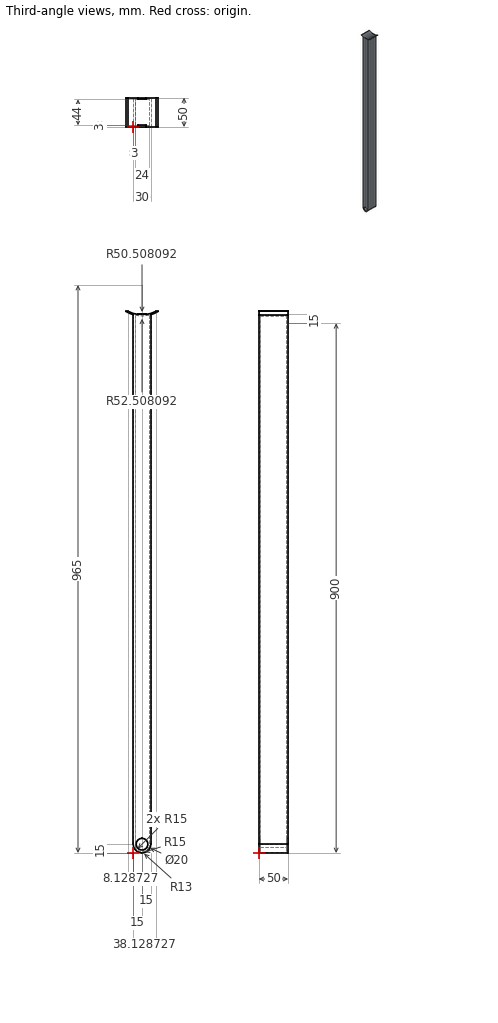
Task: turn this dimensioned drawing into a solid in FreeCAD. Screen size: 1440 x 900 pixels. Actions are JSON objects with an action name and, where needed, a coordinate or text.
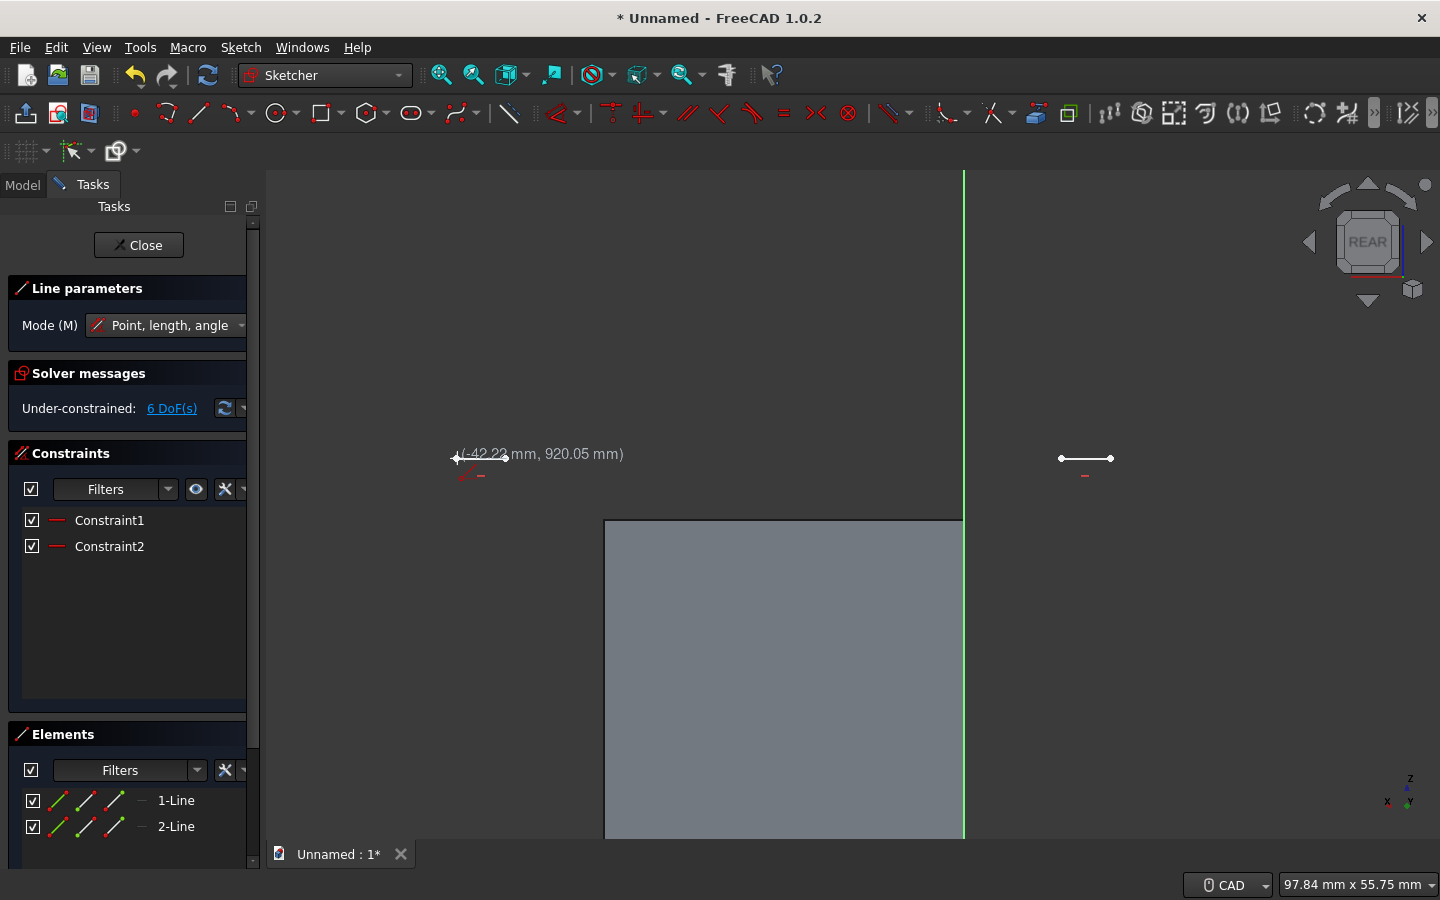
{"action": "left_click", "coordinate": [232, 114]}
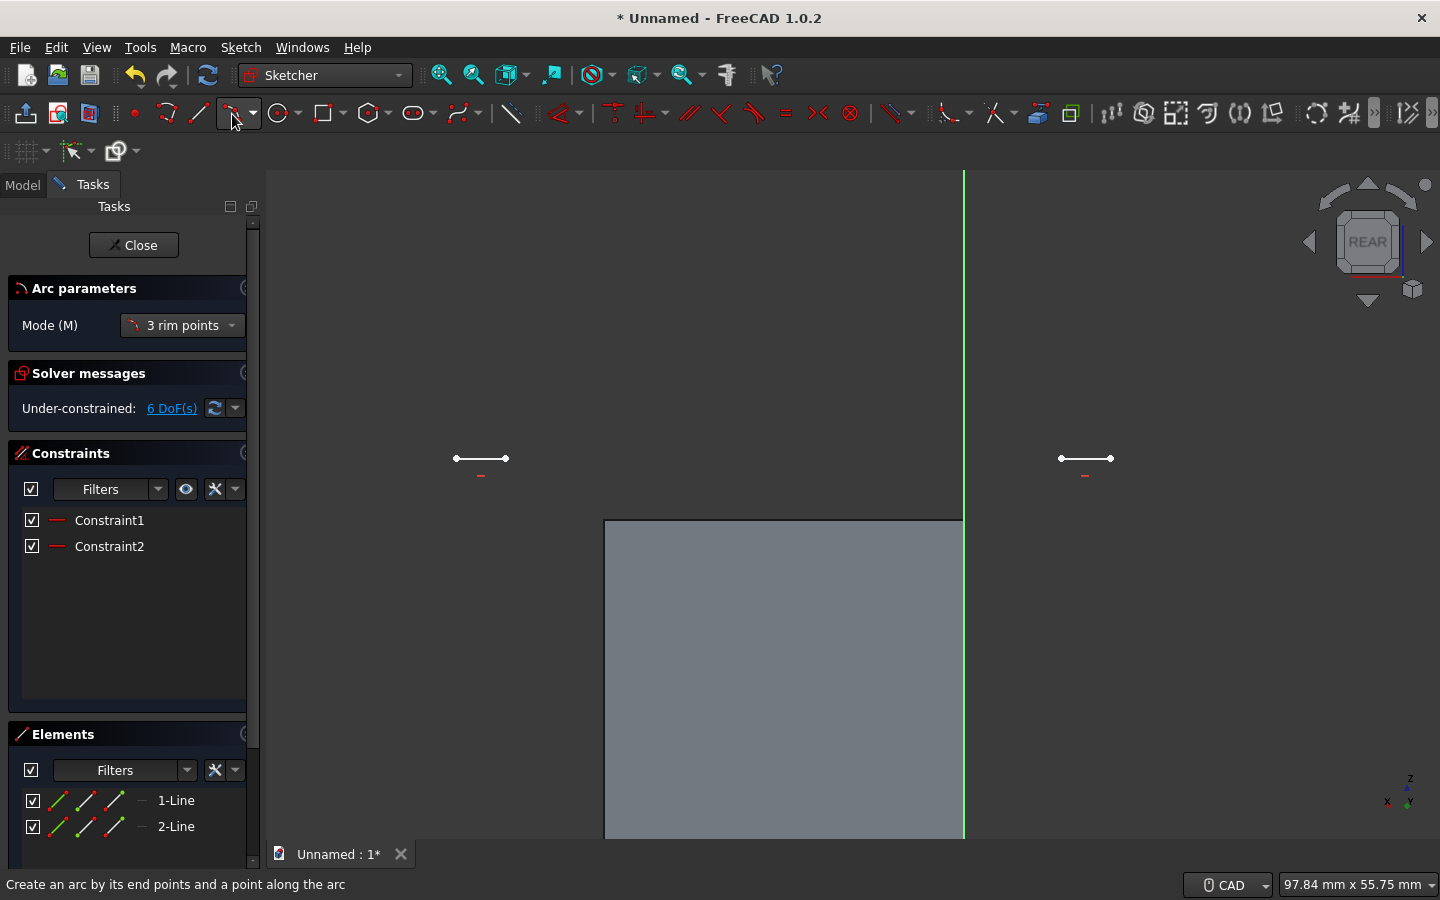
{"action": "left_click", "coordinate": [1061, 459]}
{"action": "left_click", "coordinate": [506, 459]}
{"action": "left_click", "coordinate": [784, 526]}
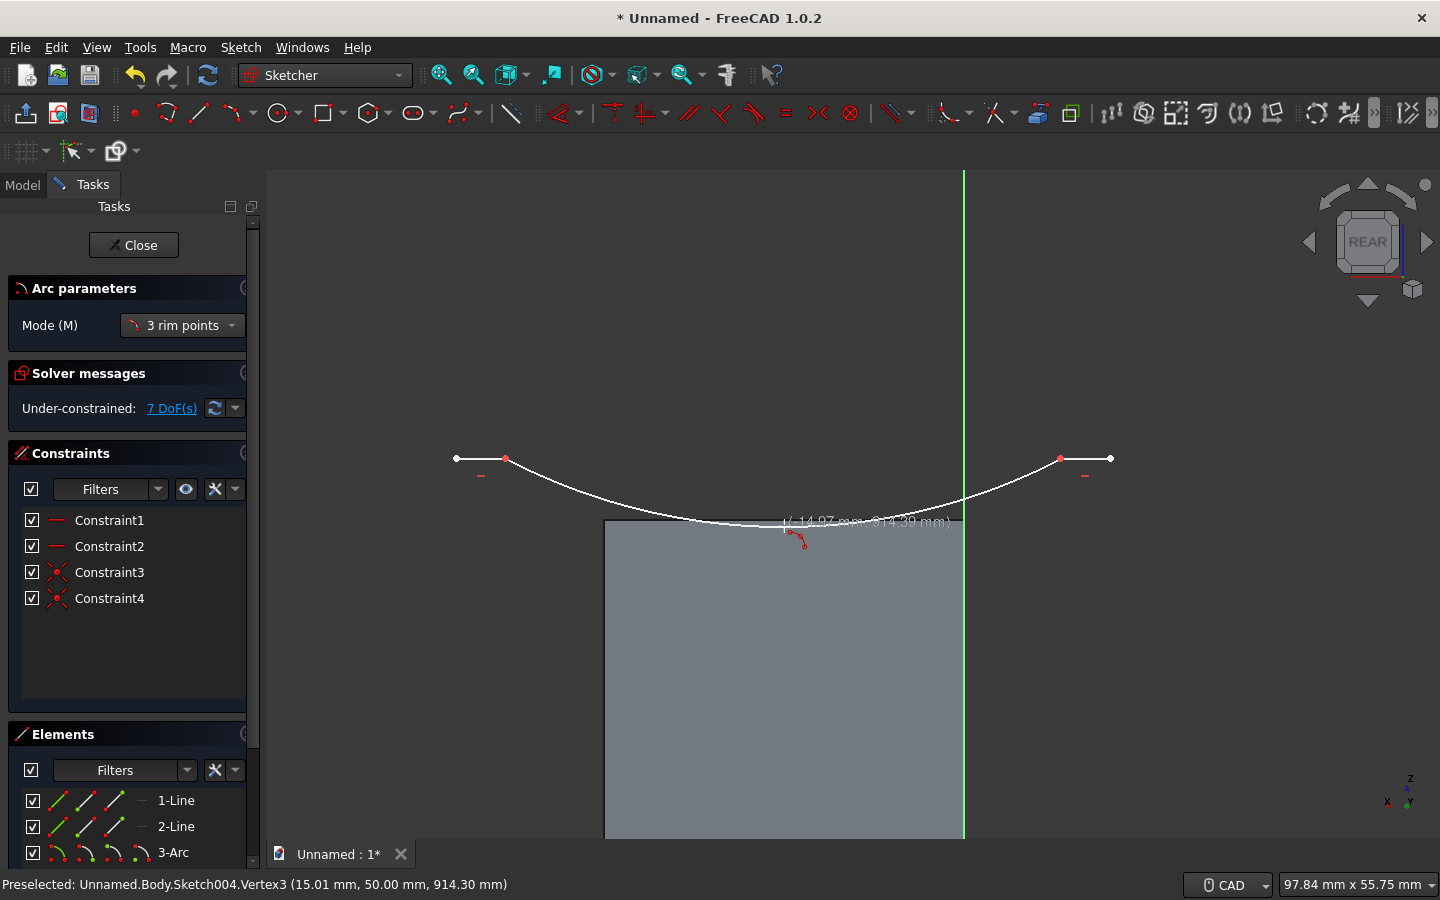
{"action": "left_click", "coordinate": [457, 459]}
{"action": "left_click", "coordinate": [1110, 459]}
{"action": "left_click", "coordinate": [784, 550]}
{"action": "key", "text": "Escape"}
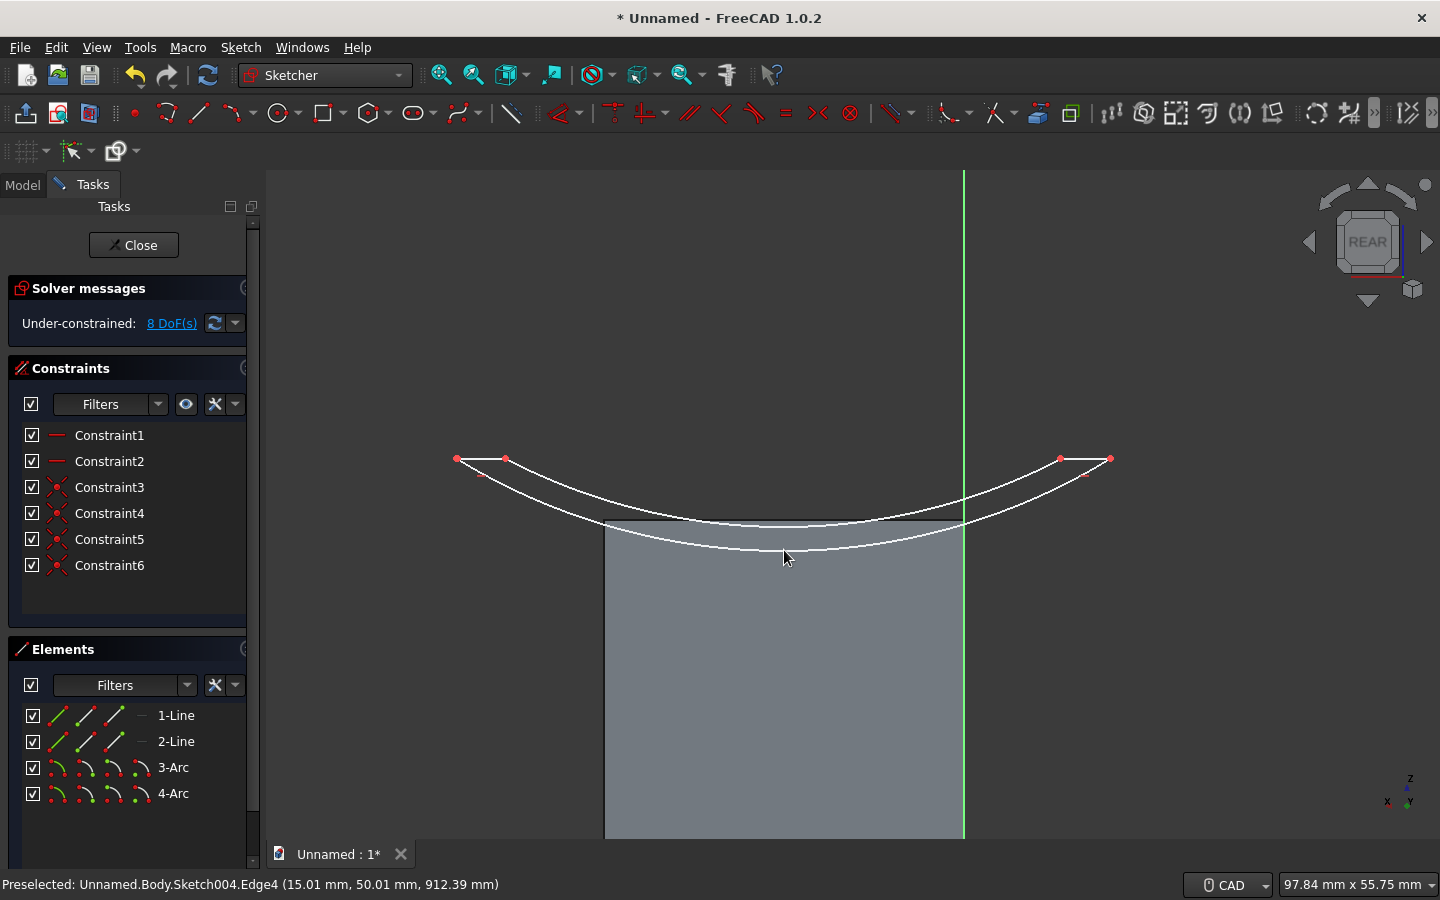
{"action": "left_click", "coordinate": [669, 516]}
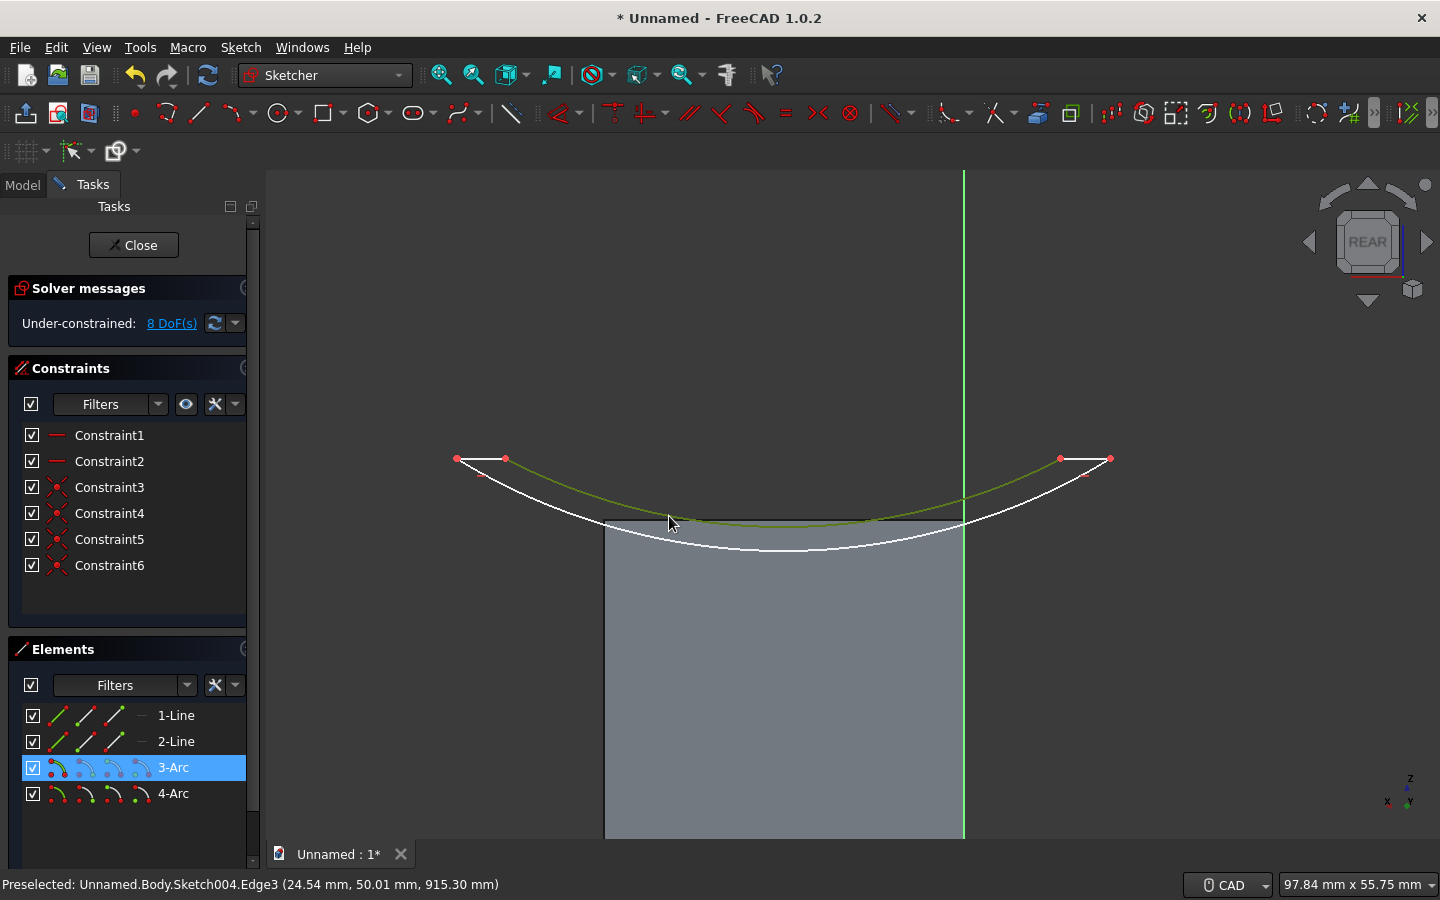
{"action": "left_click", "coordinate": [647, 536]}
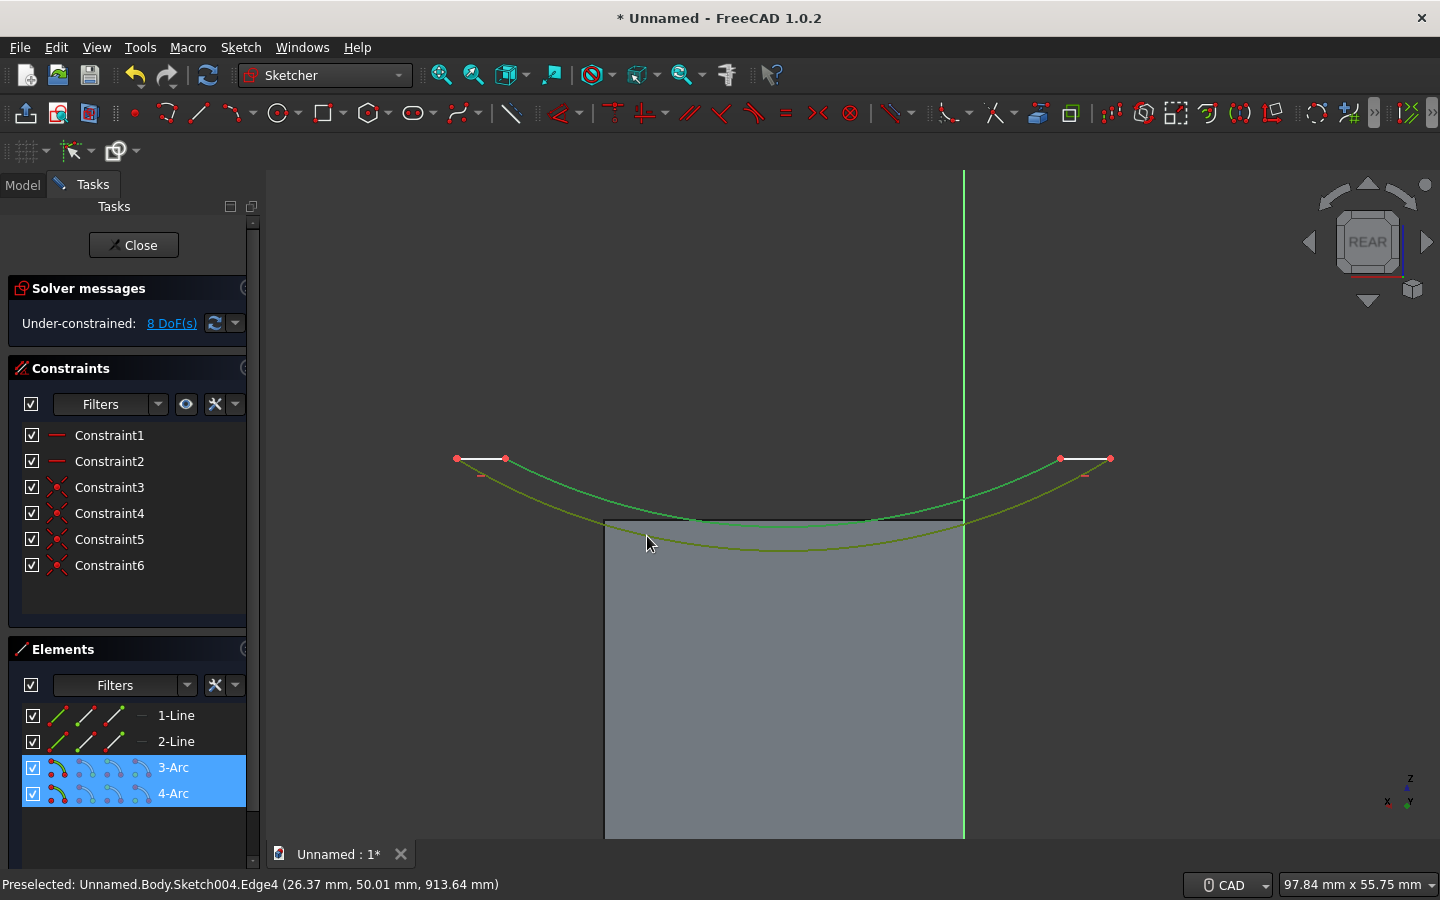
{"action": "left_click", "coordinate": [614, 114]}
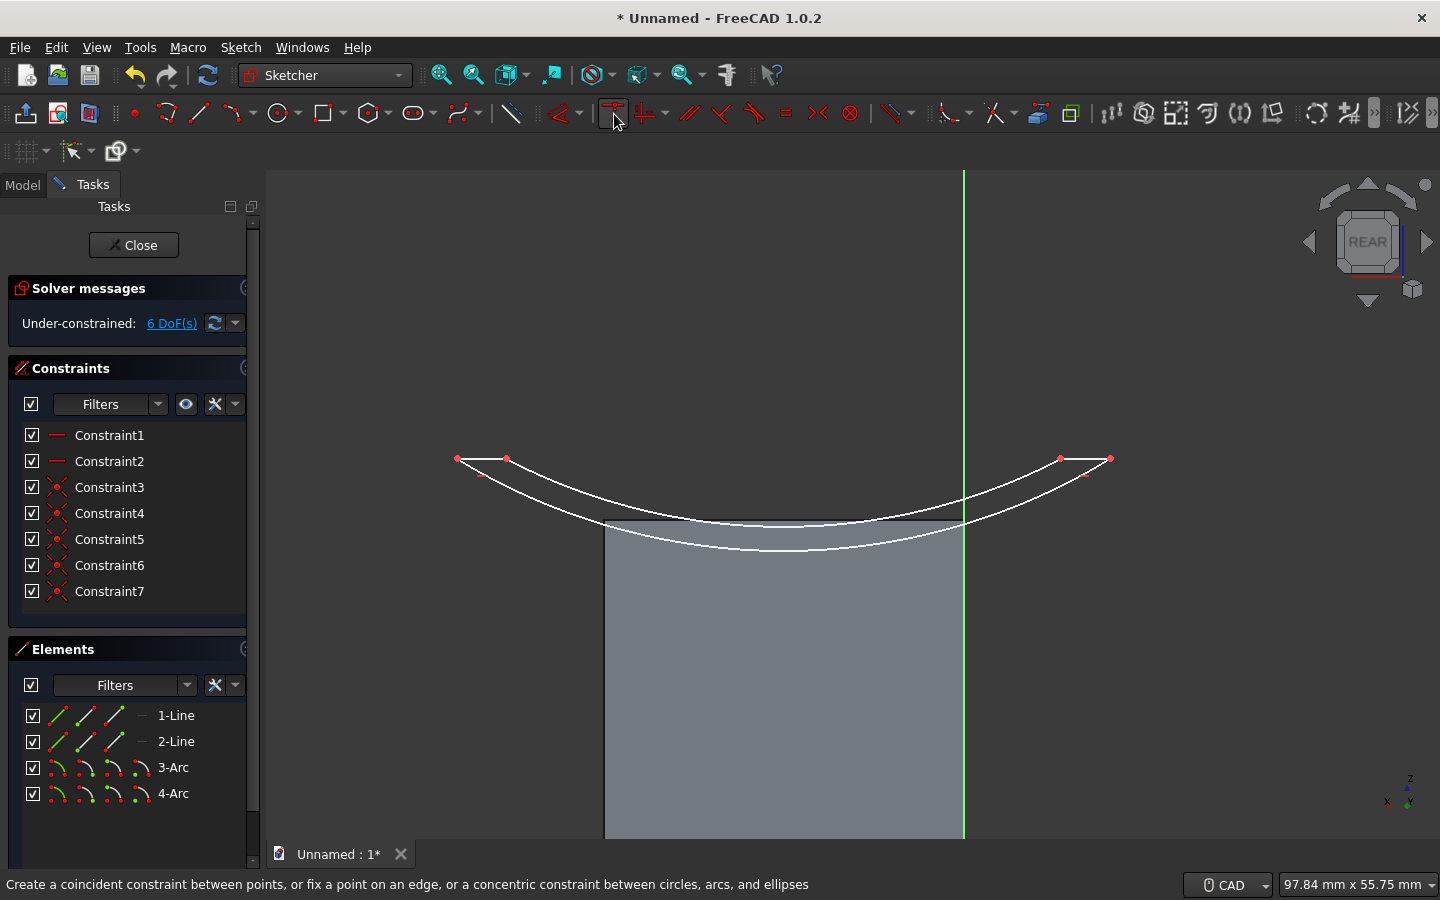
{"action": "left_click", "coordinate": [558, 114]}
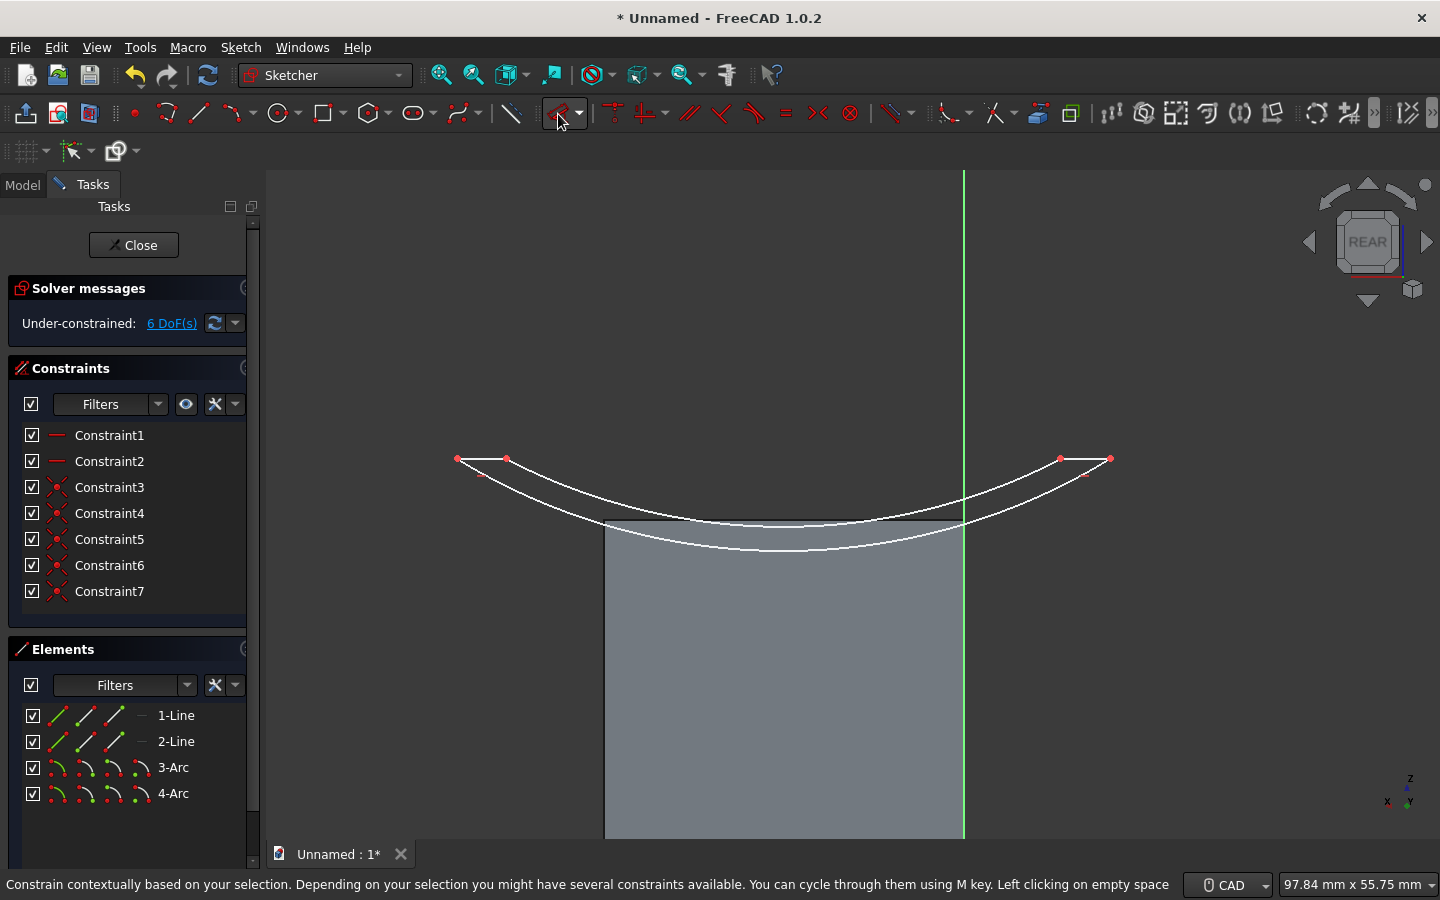
{"action": "left_click", "coordinate": [669, 516]}
{"action": "left_click", "coordinate": [380, 413]}